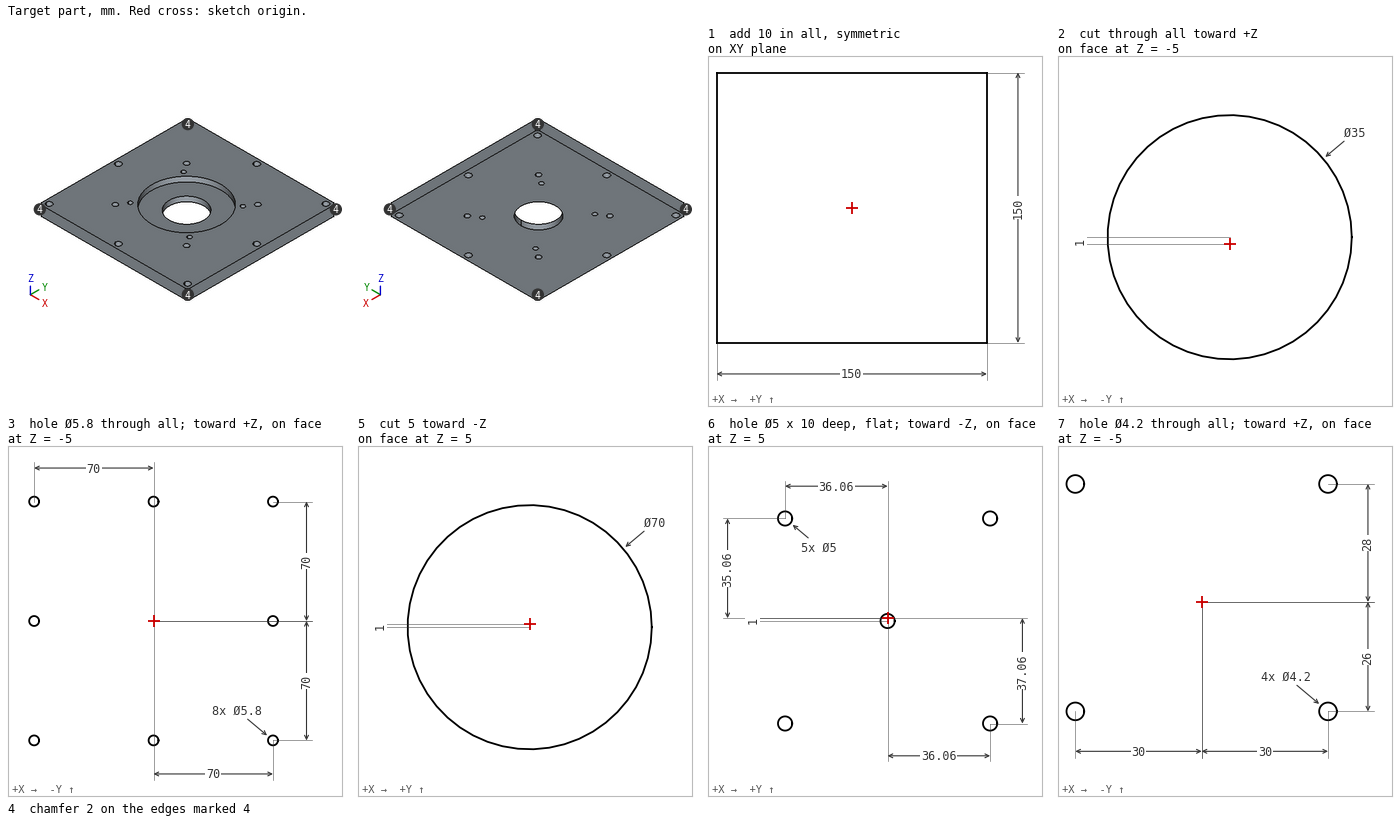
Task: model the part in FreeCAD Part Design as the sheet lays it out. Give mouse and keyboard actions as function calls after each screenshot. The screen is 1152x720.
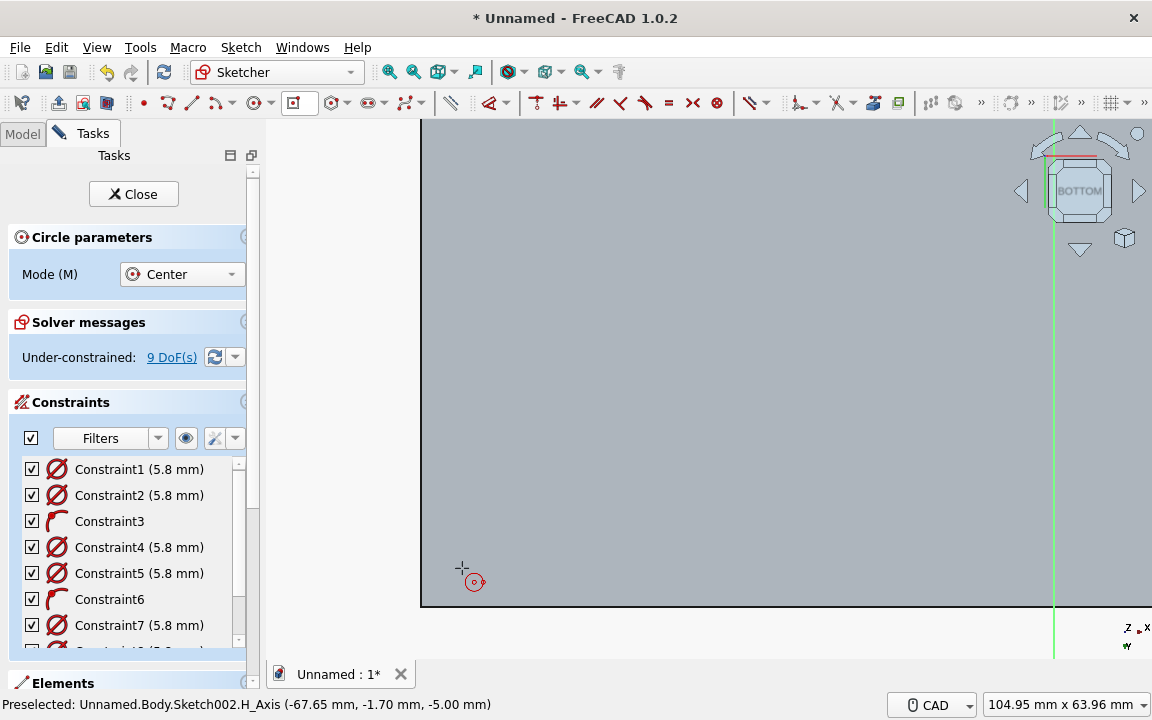
click(463, 565)
move(480, 548)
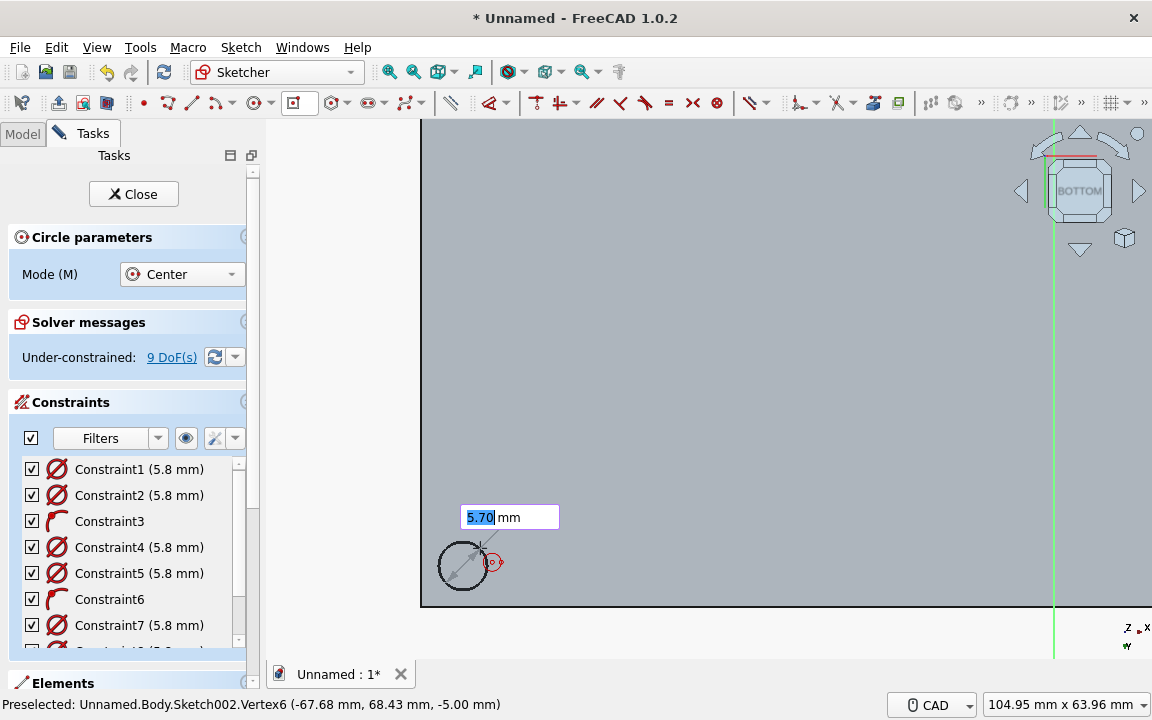
text(5.8)
key(Return)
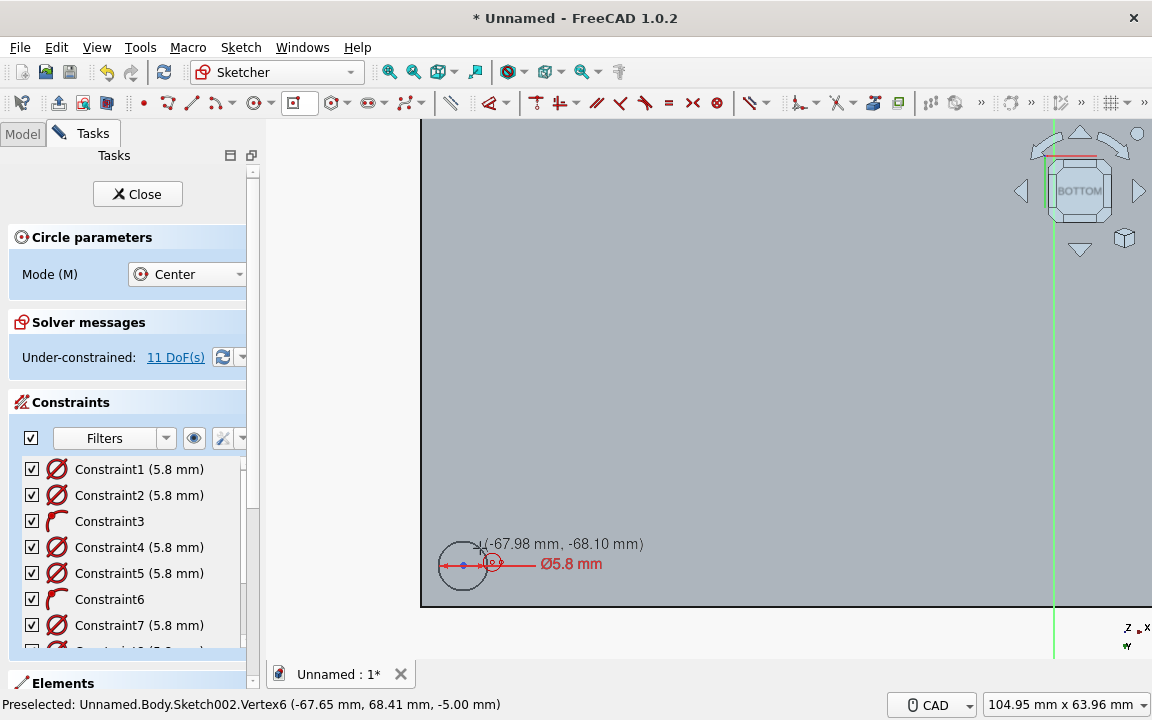
scroll(462, 568, down, 6)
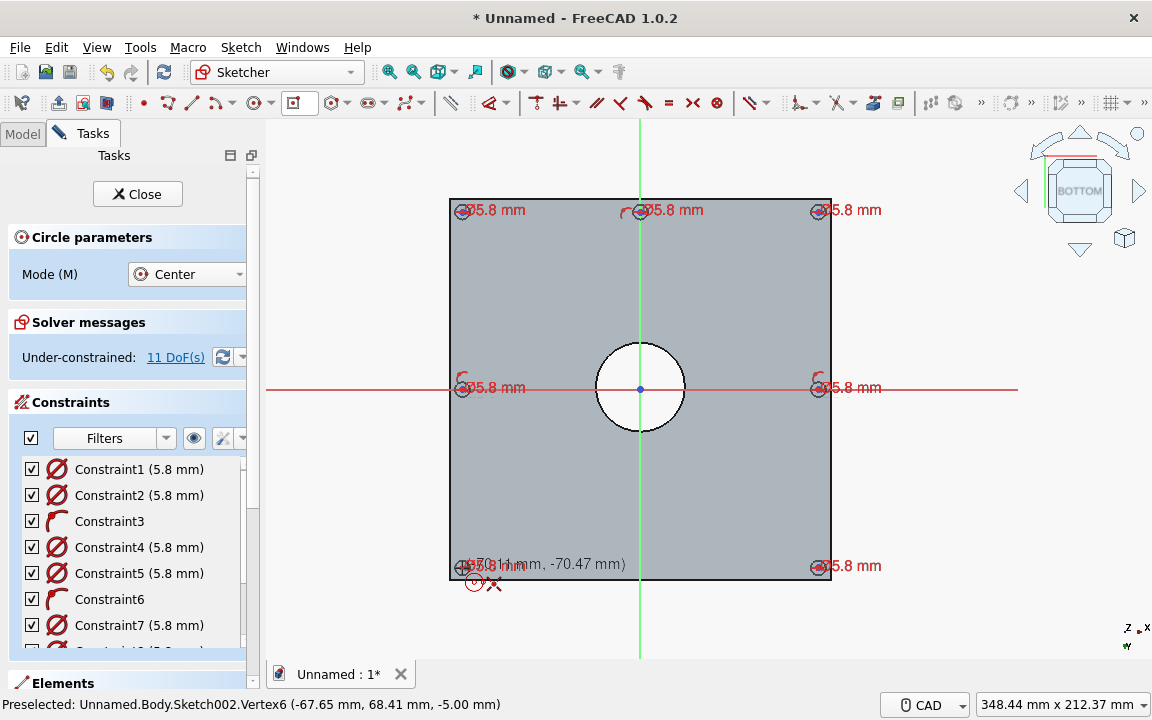
scroll(640, 568, up, 6)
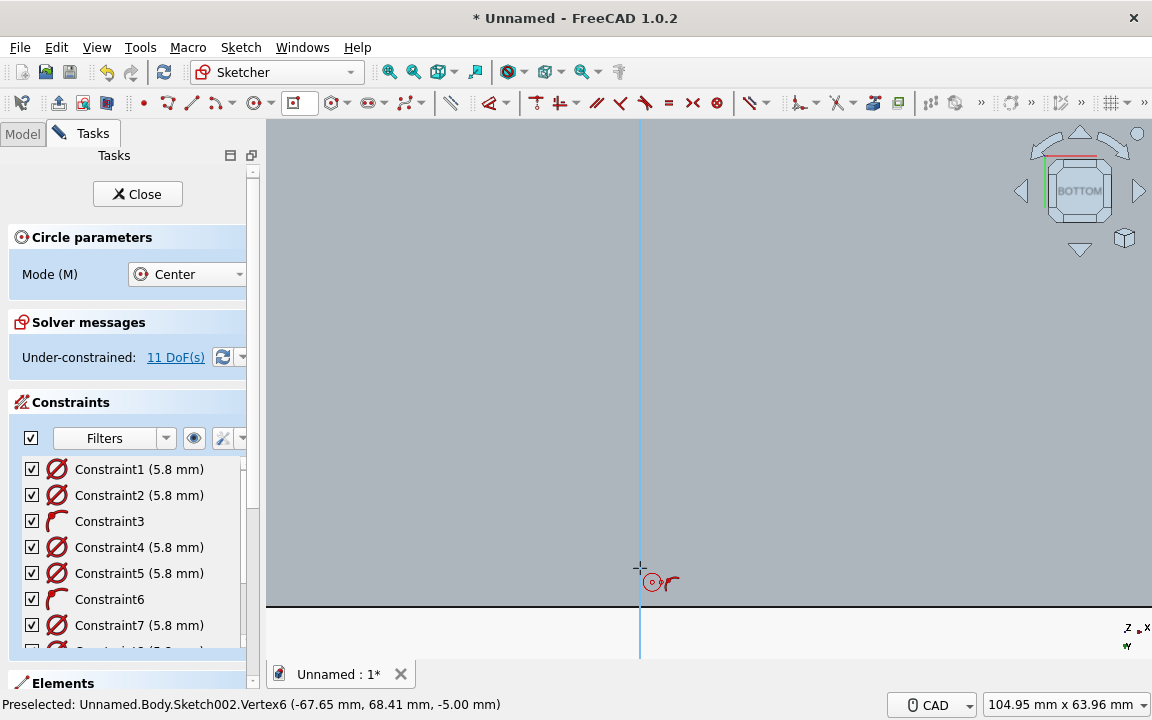
click(640, 565)
move(658, 548)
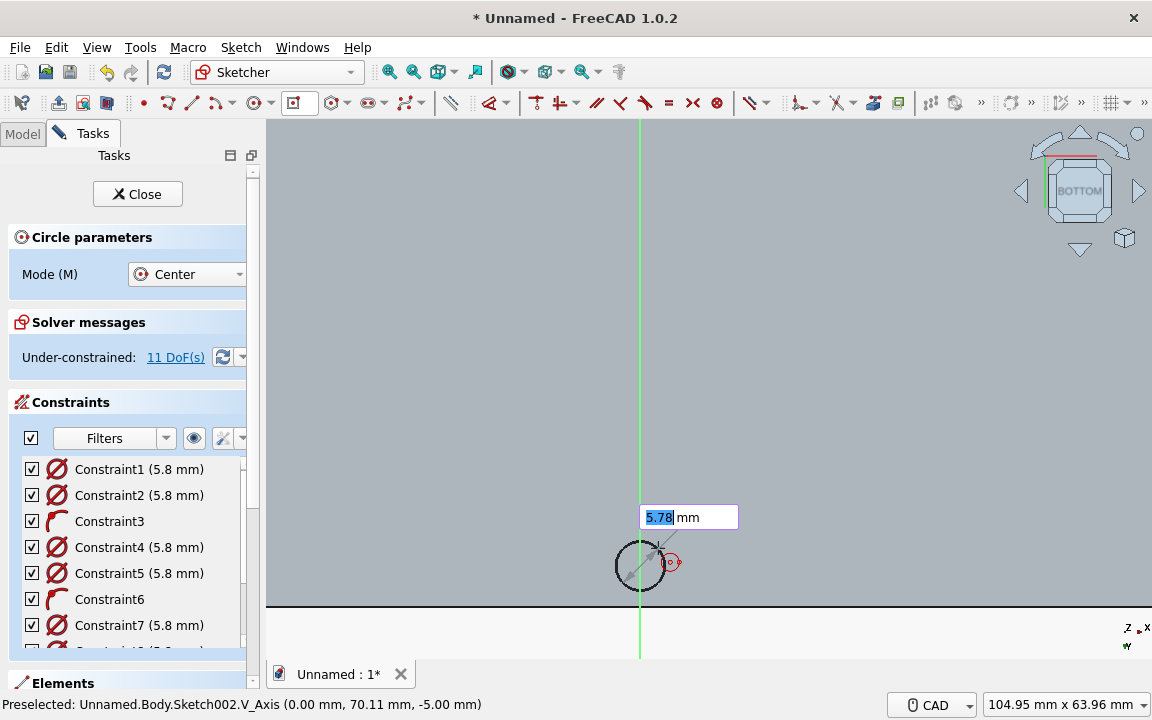
text(5.8)
key(Return)
key(Escape)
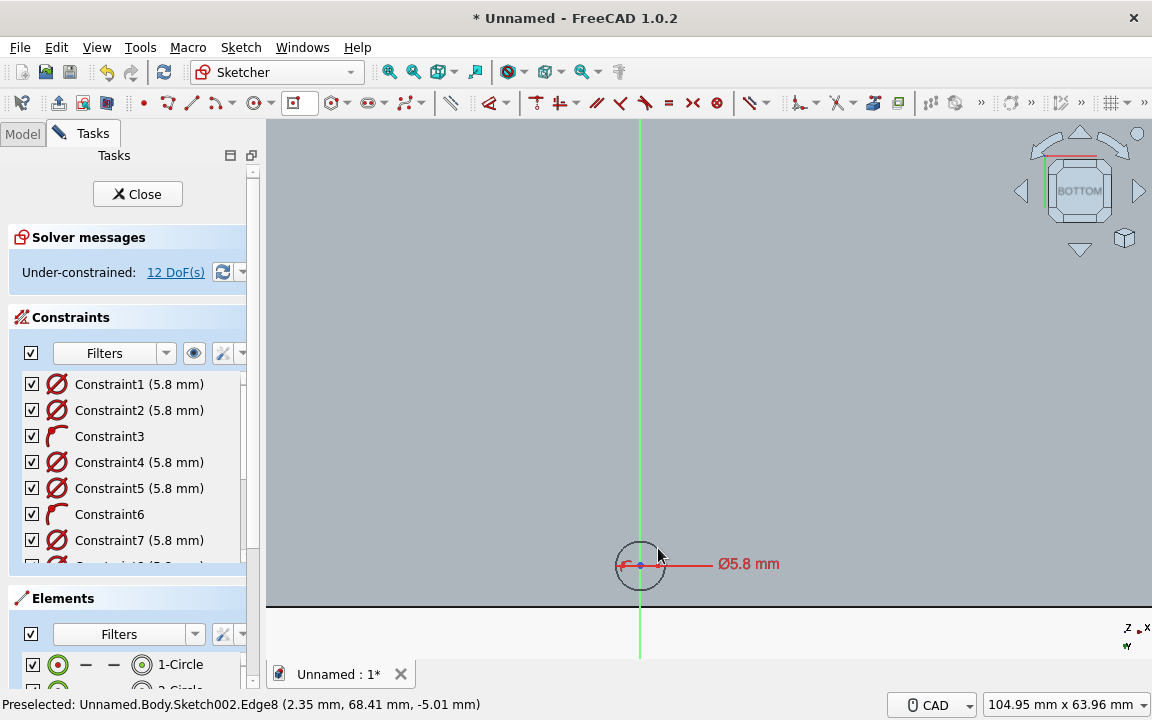
scroll(641, 568, down, 6)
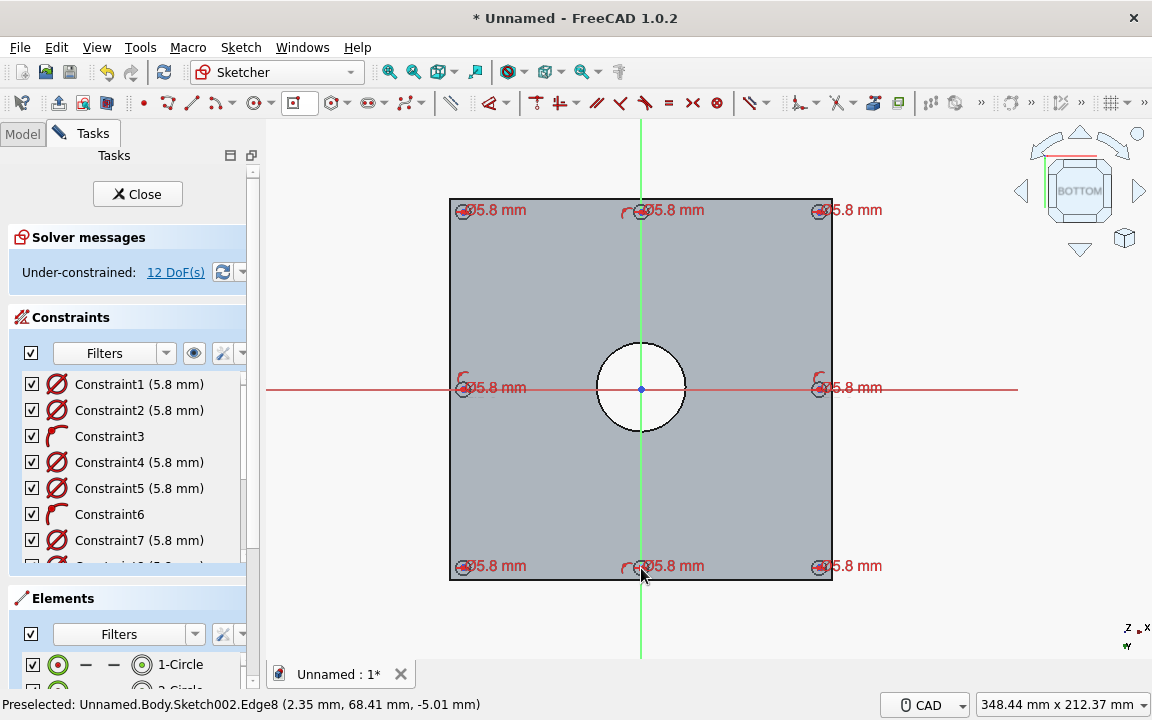
click(819, 568)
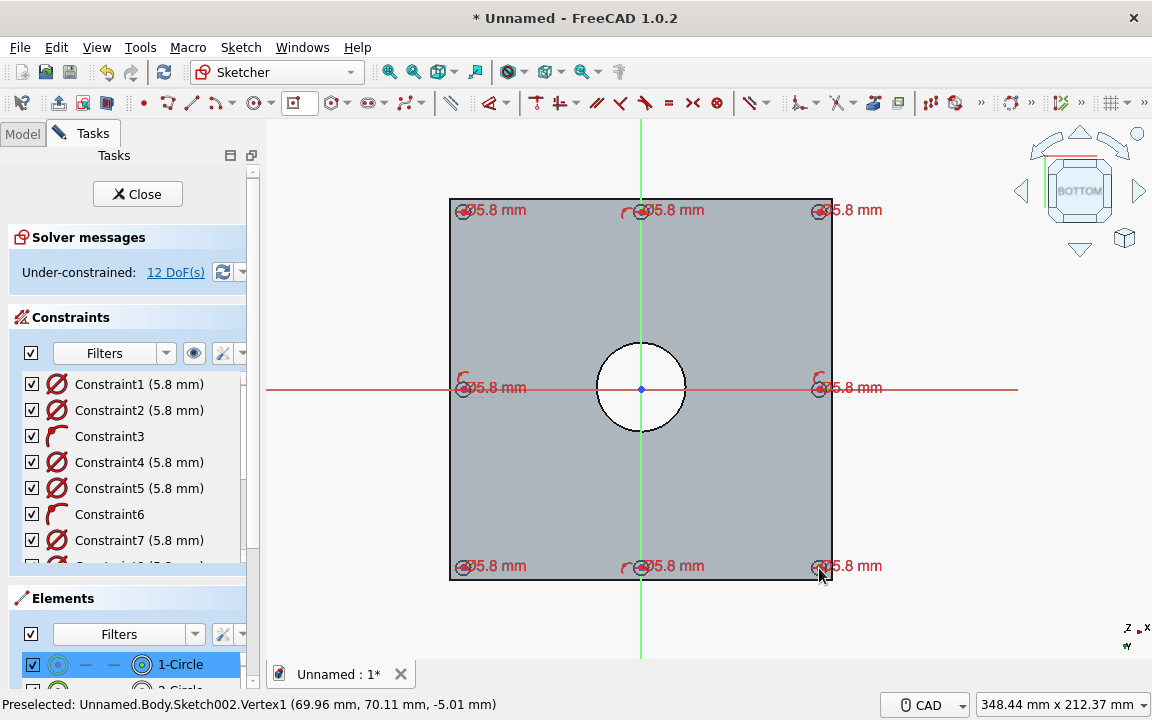
click(819, 390)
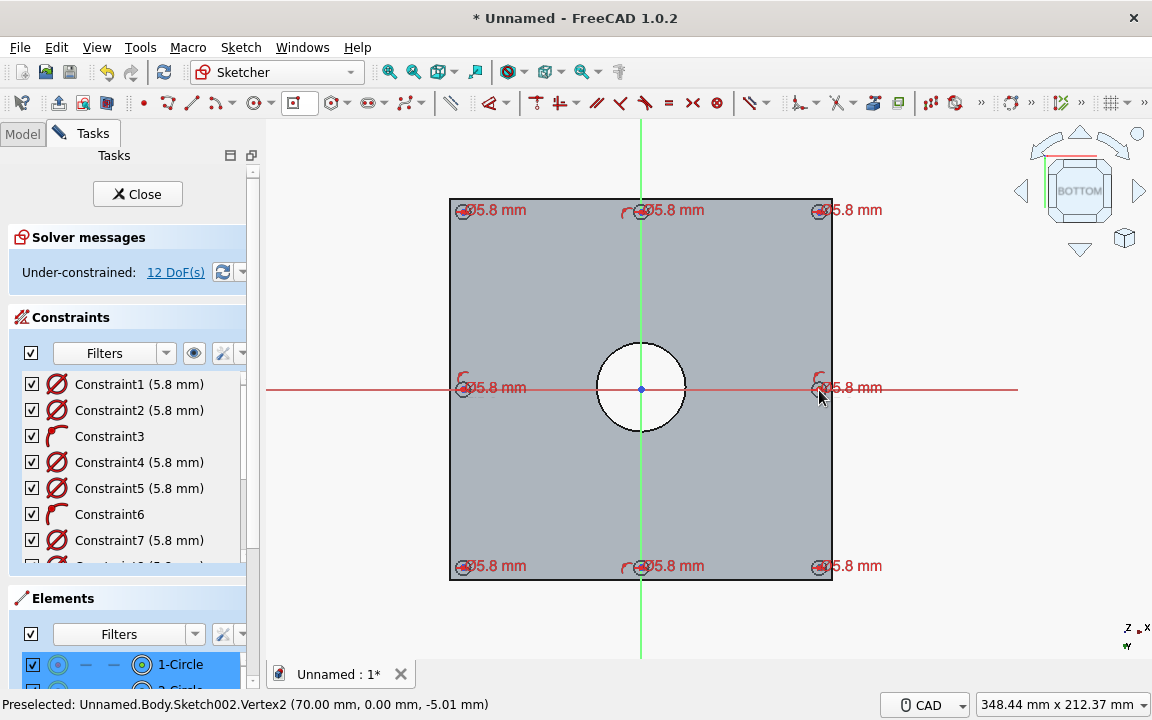
key(v)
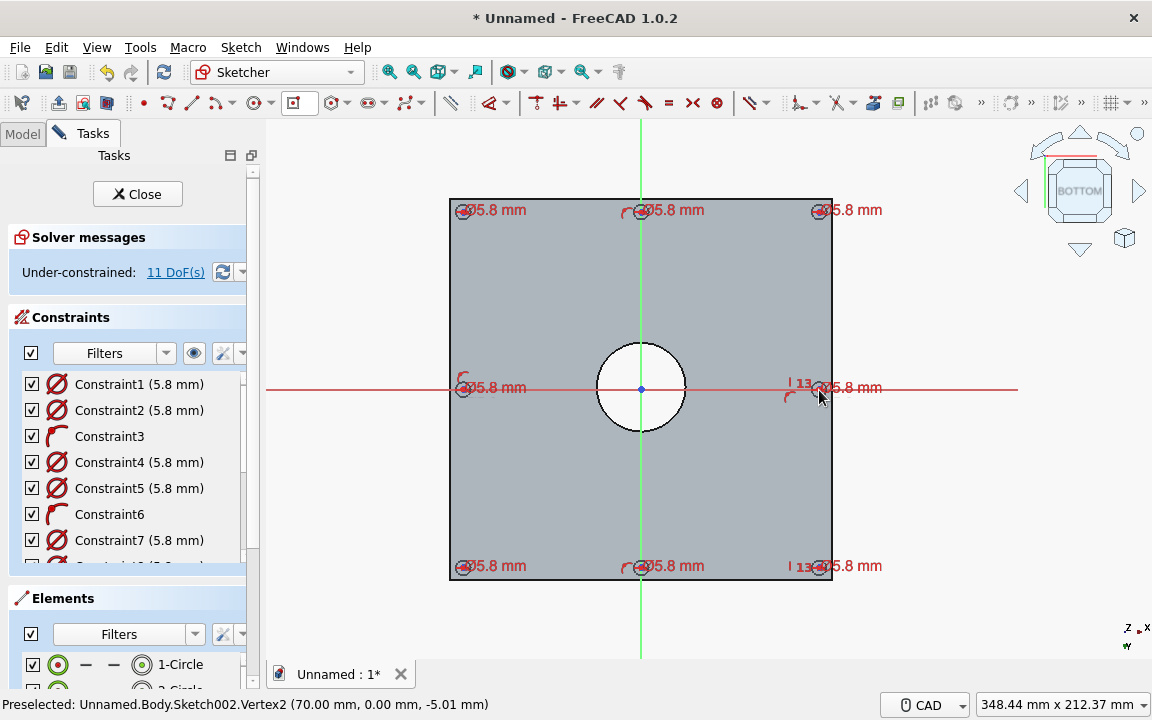
click(819, 390)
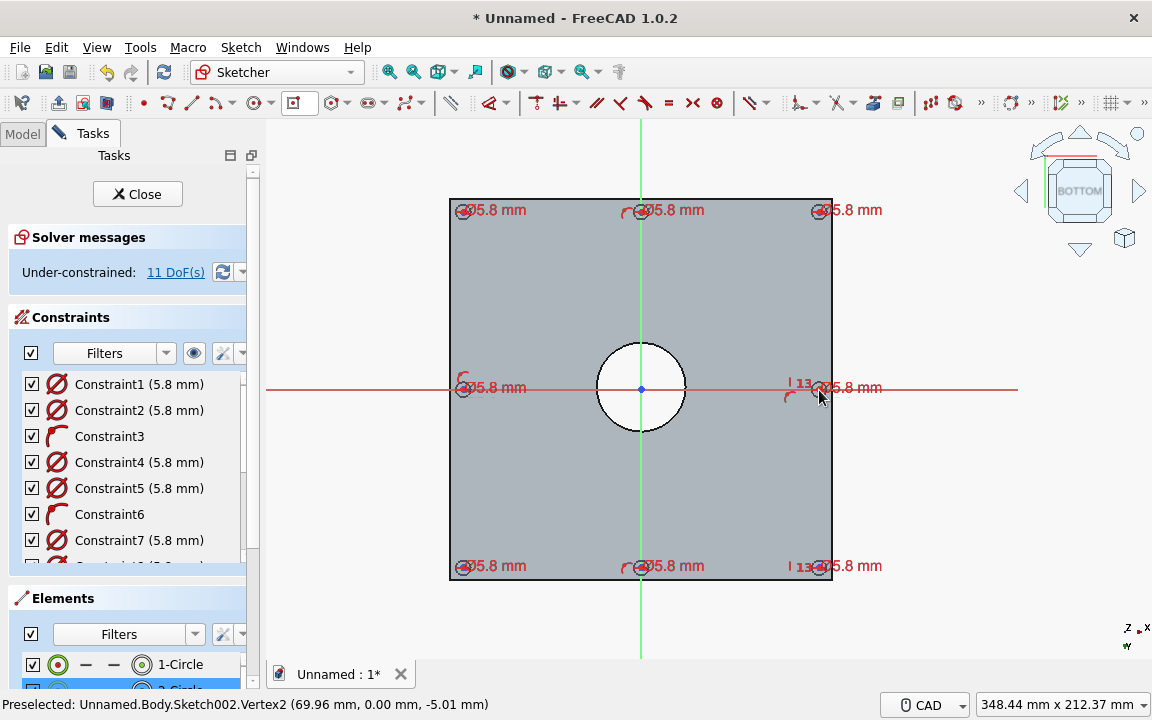
click(819, 212)